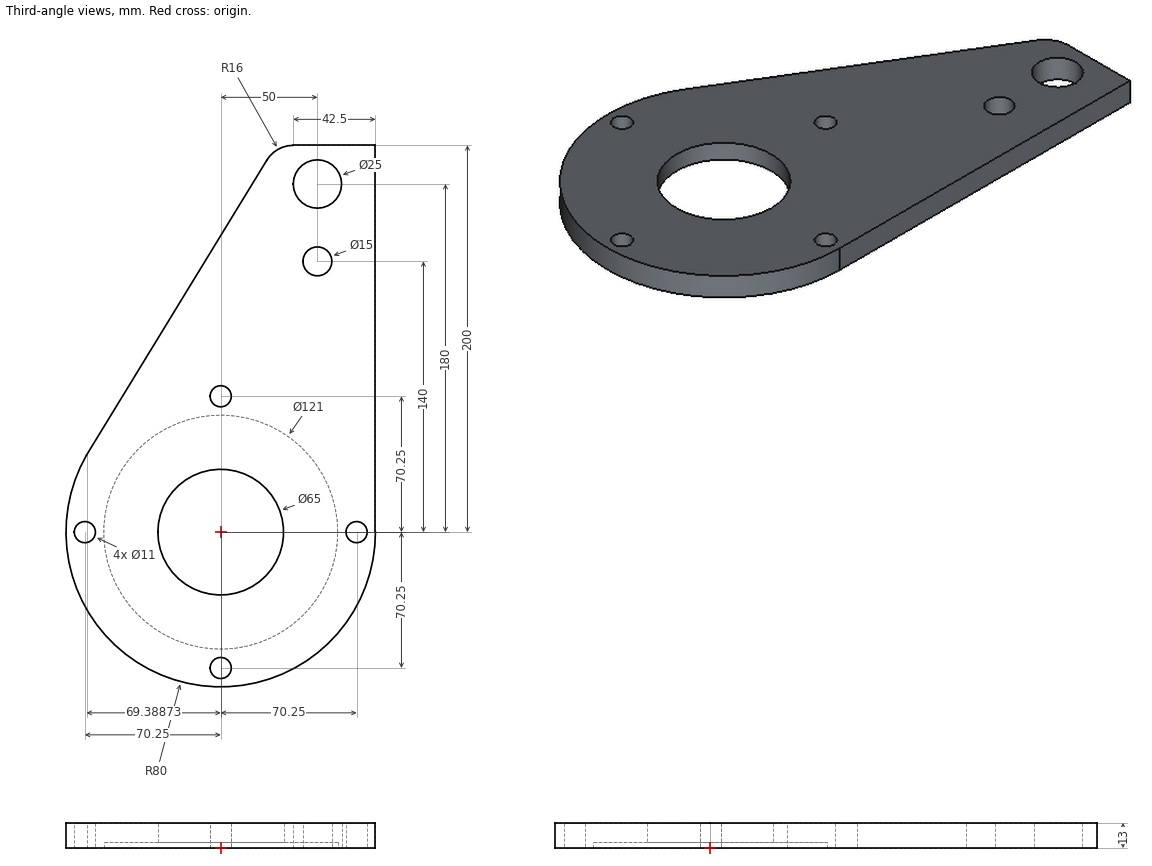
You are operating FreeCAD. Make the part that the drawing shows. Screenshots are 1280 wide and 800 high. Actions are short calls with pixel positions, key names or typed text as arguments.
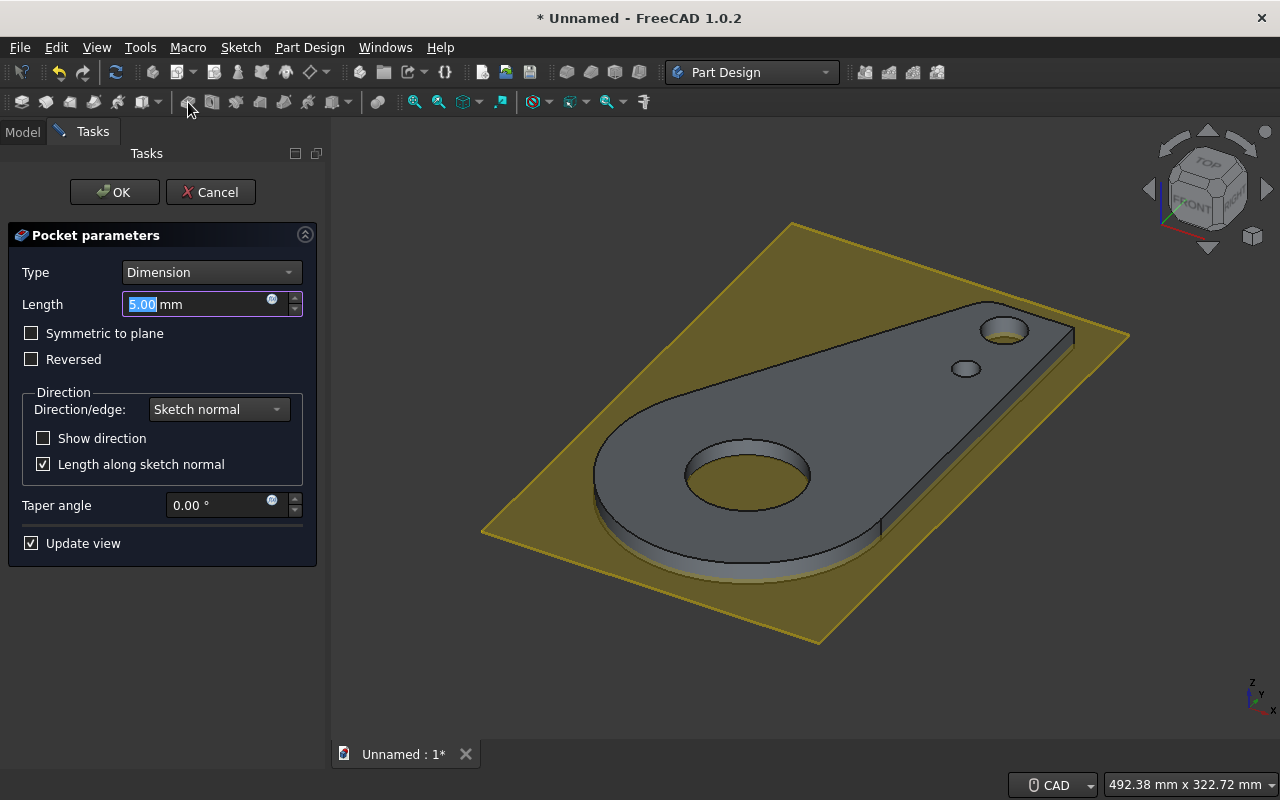
click(212, 272)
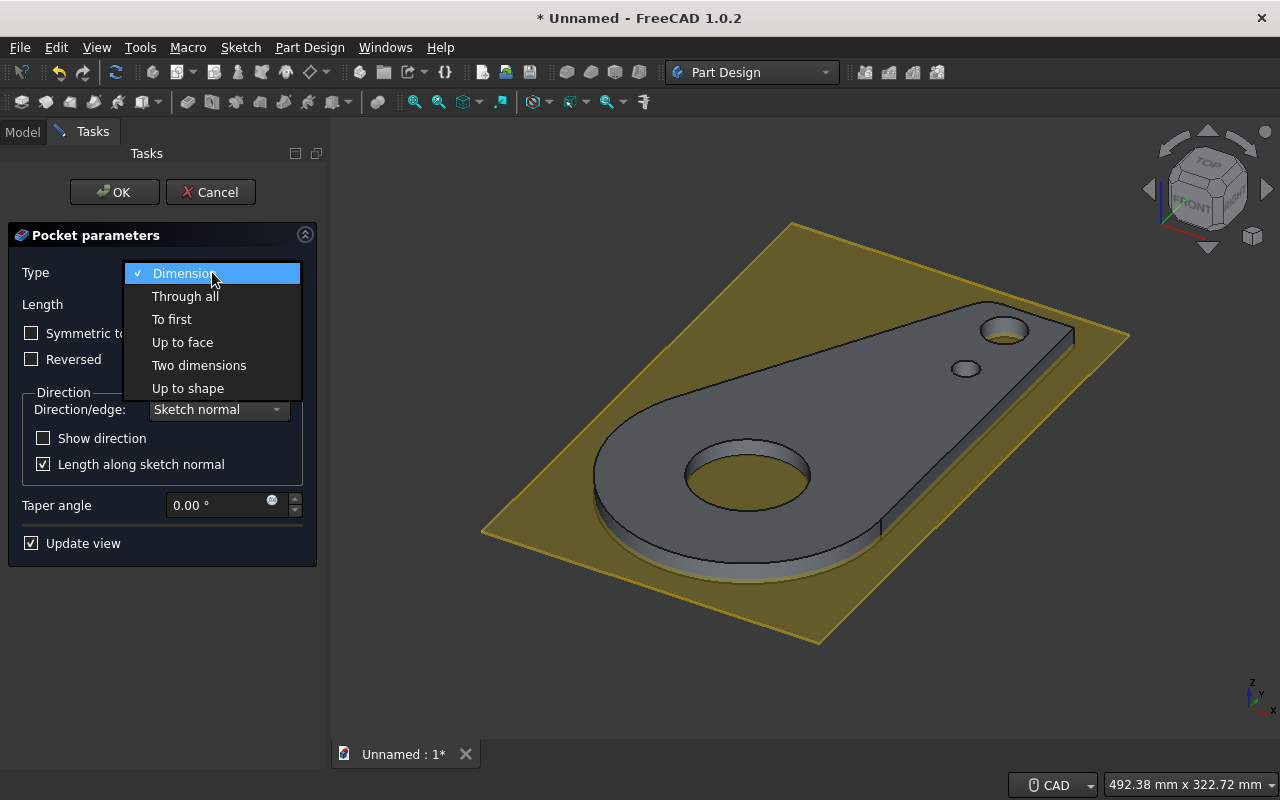
click(212, 296)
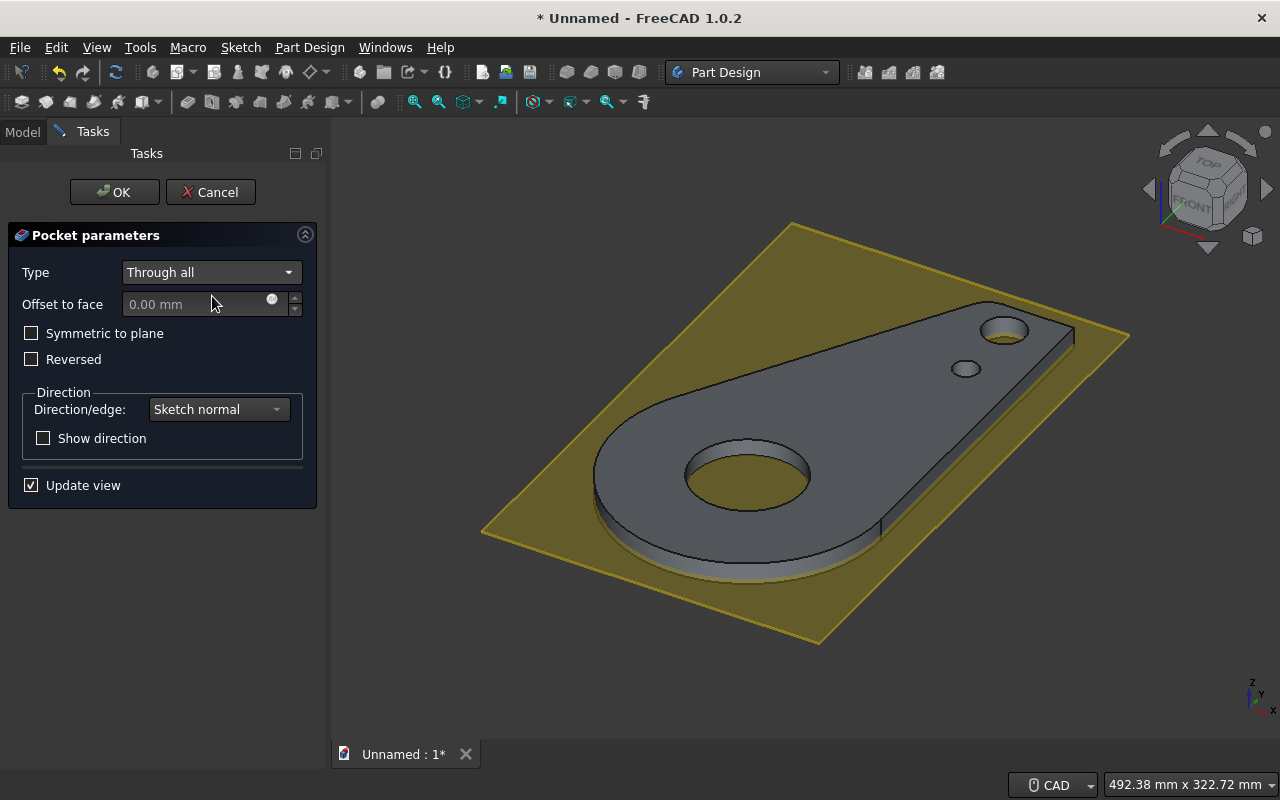
click(115, 192)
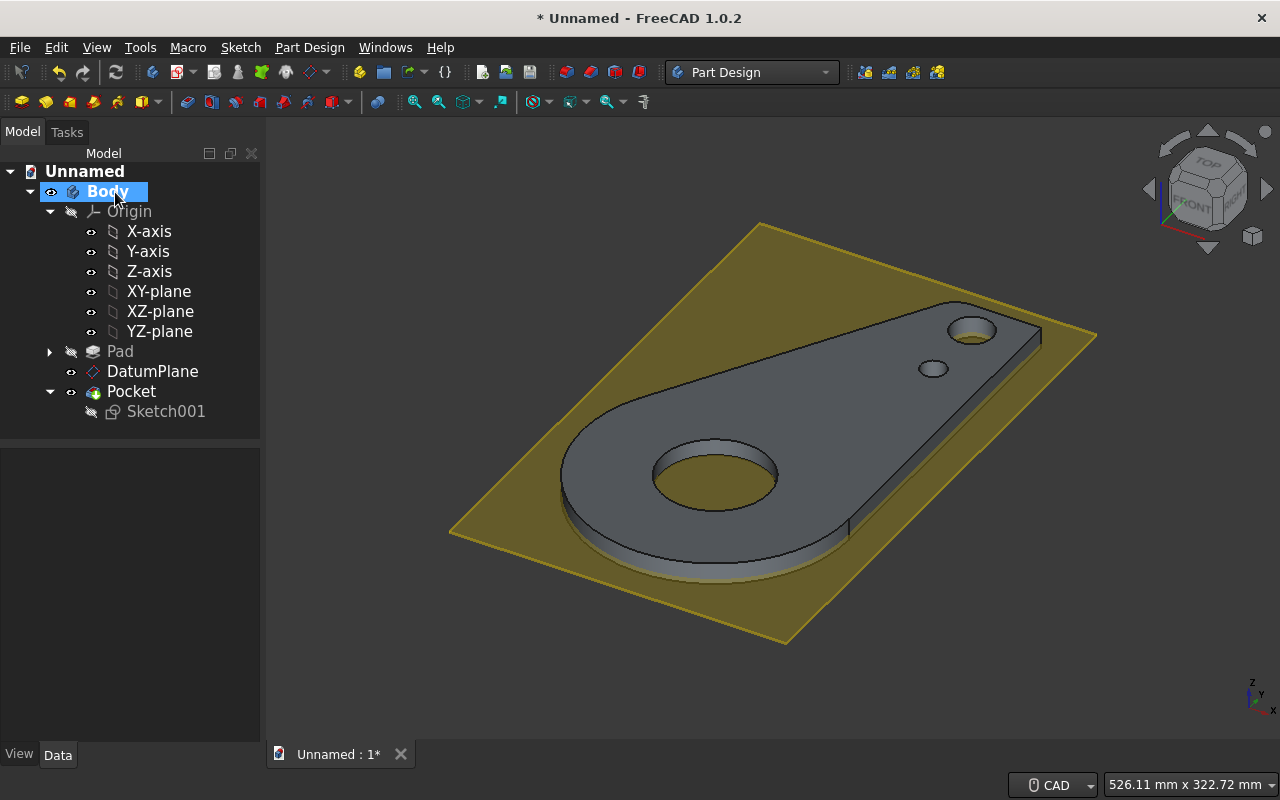
click(116, 372)
key(space)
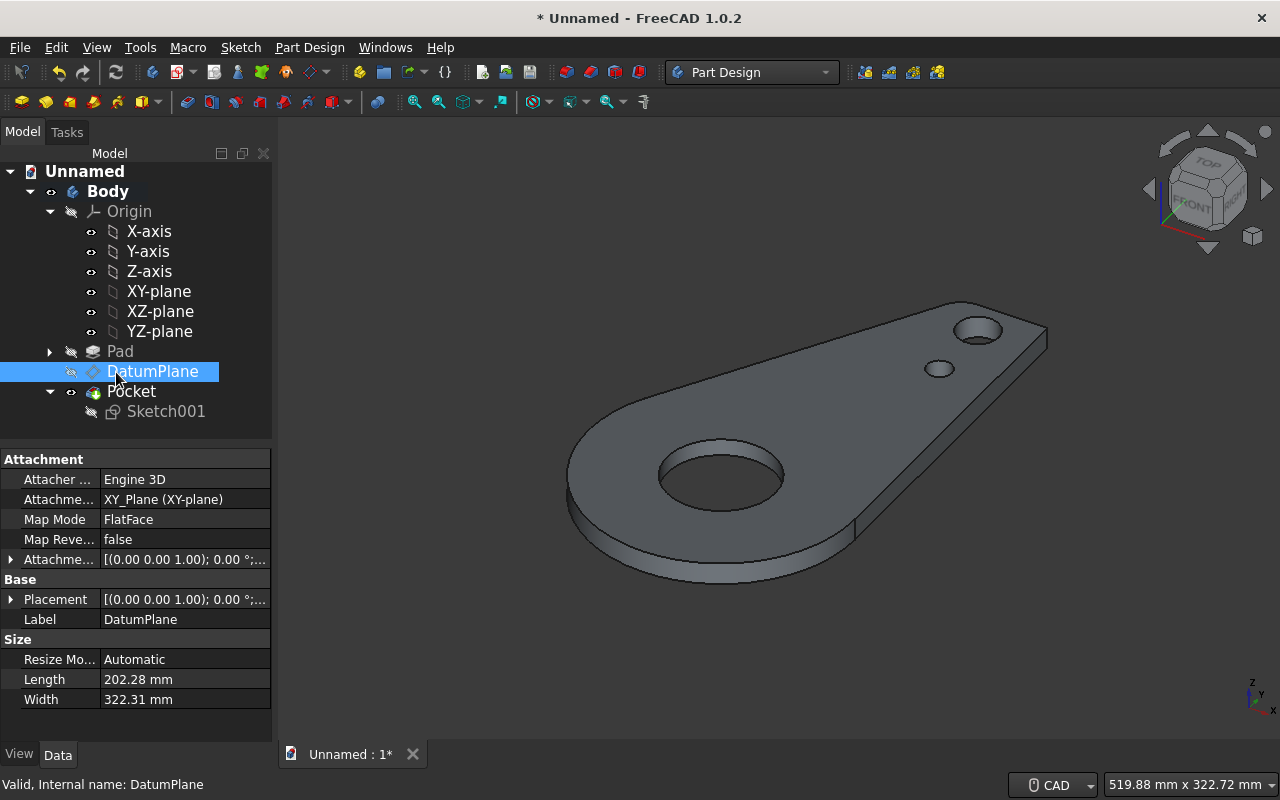
key(5)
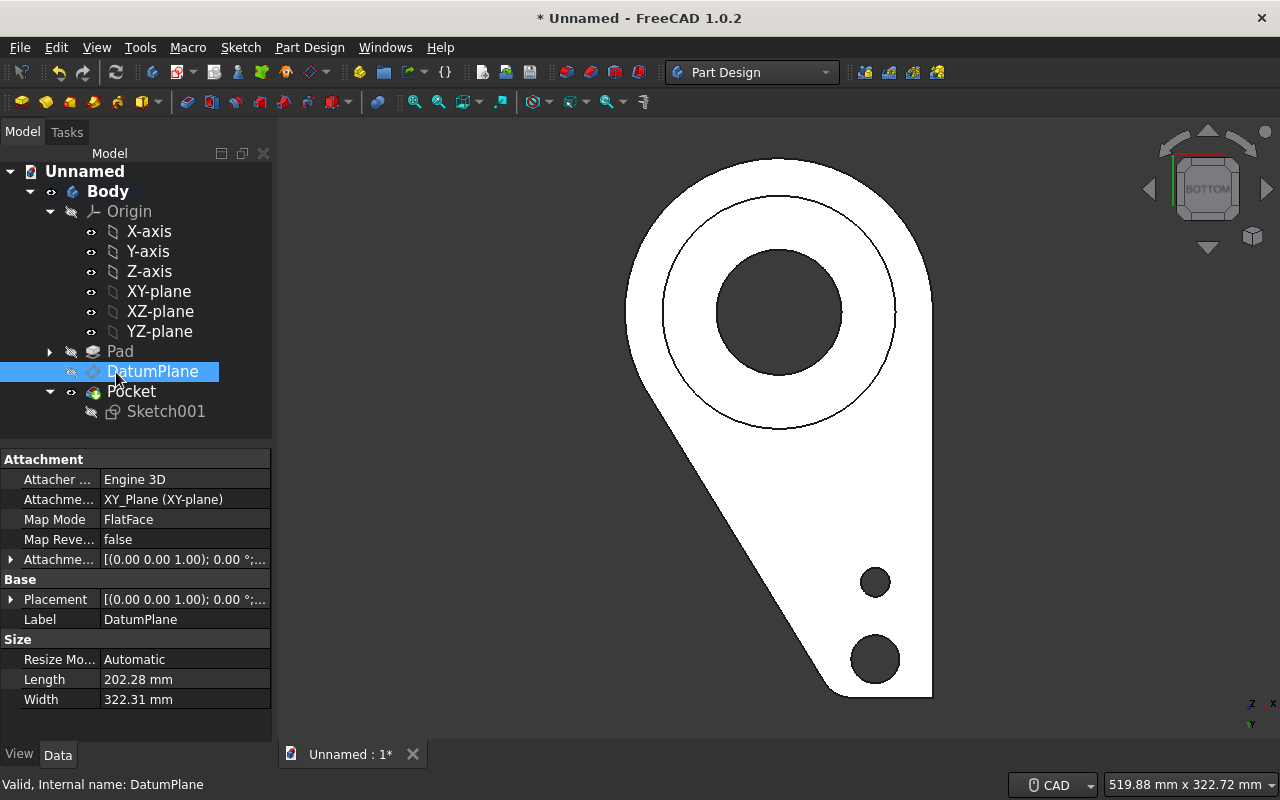
click(823, 504)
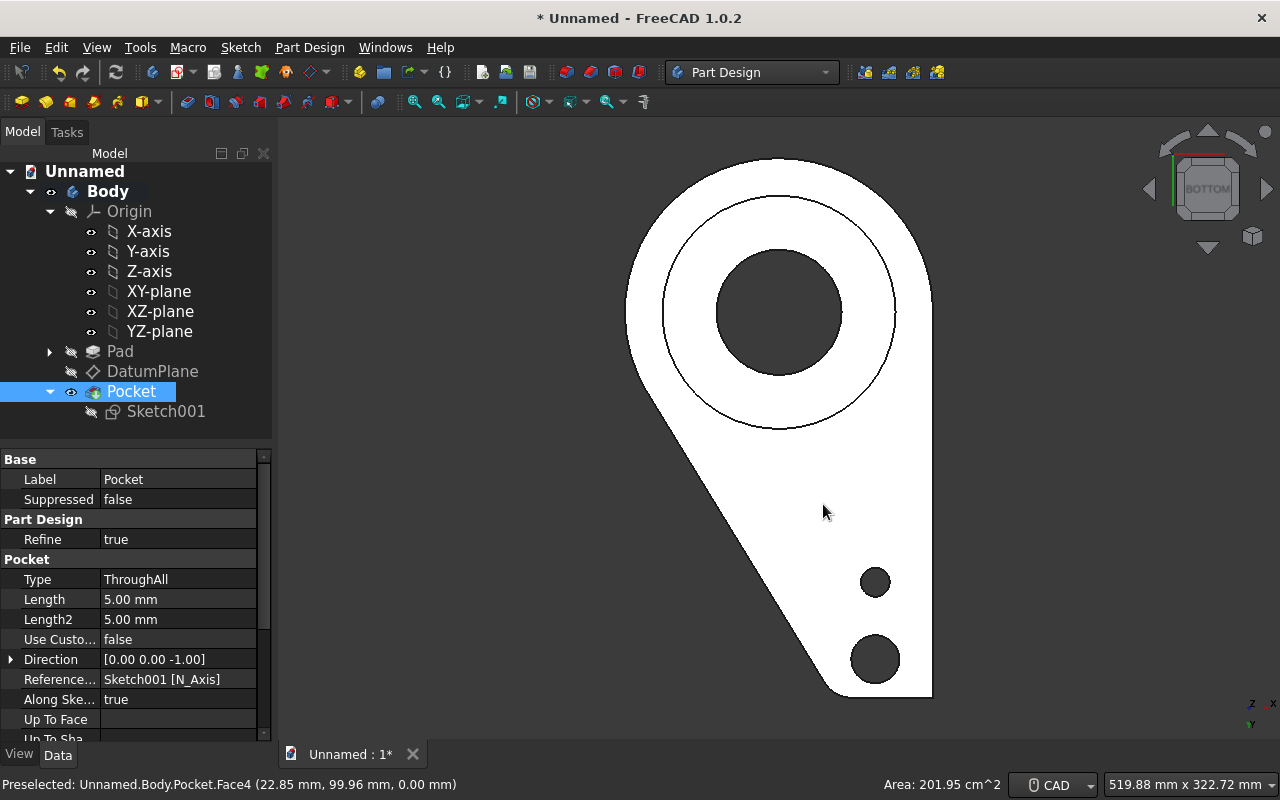
click(178, 72)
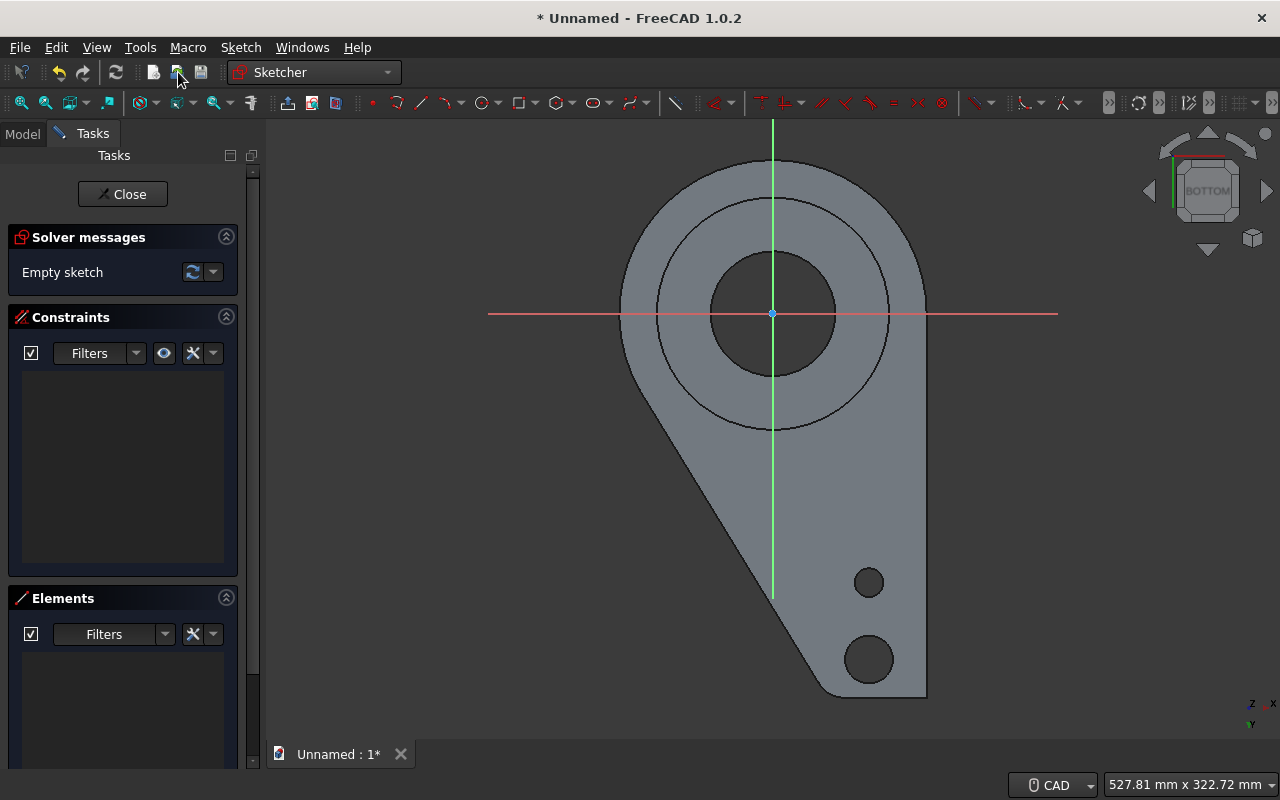
scroll(912, 147, up, 2)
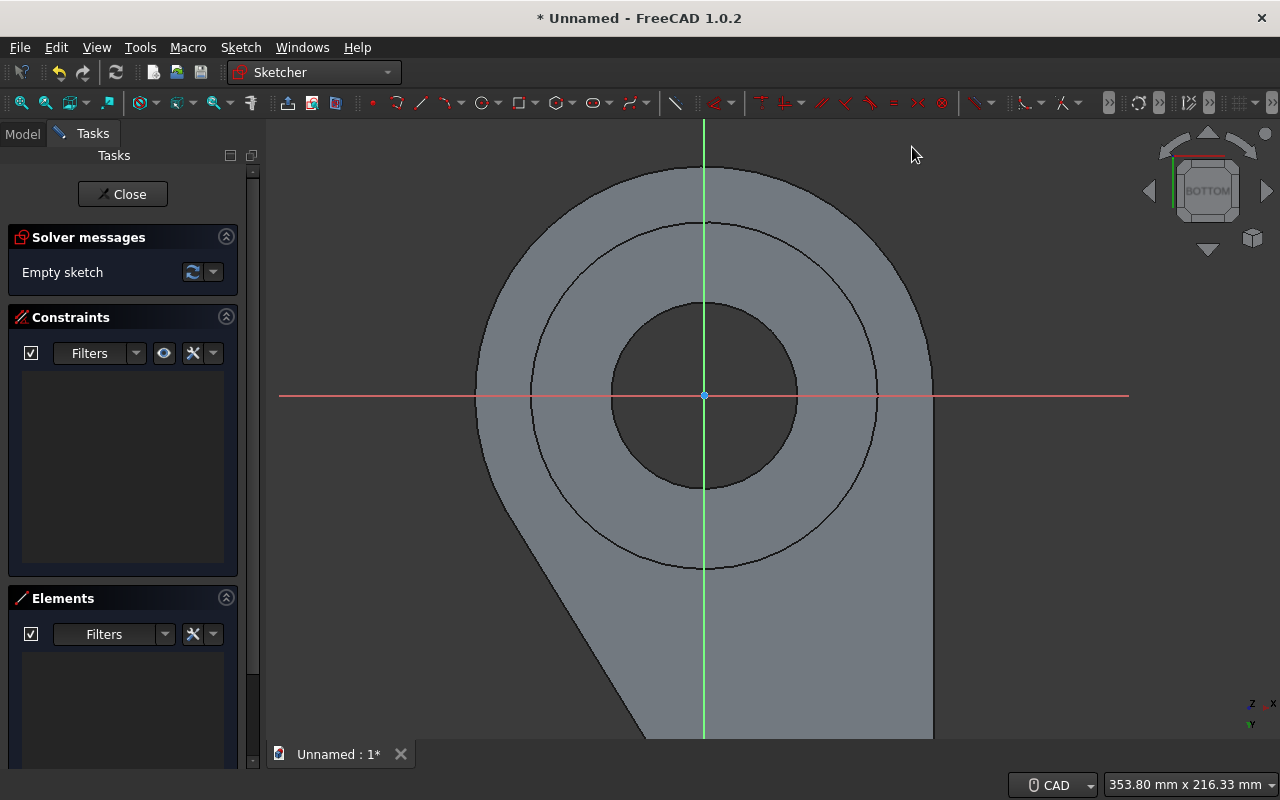
click(482, 104)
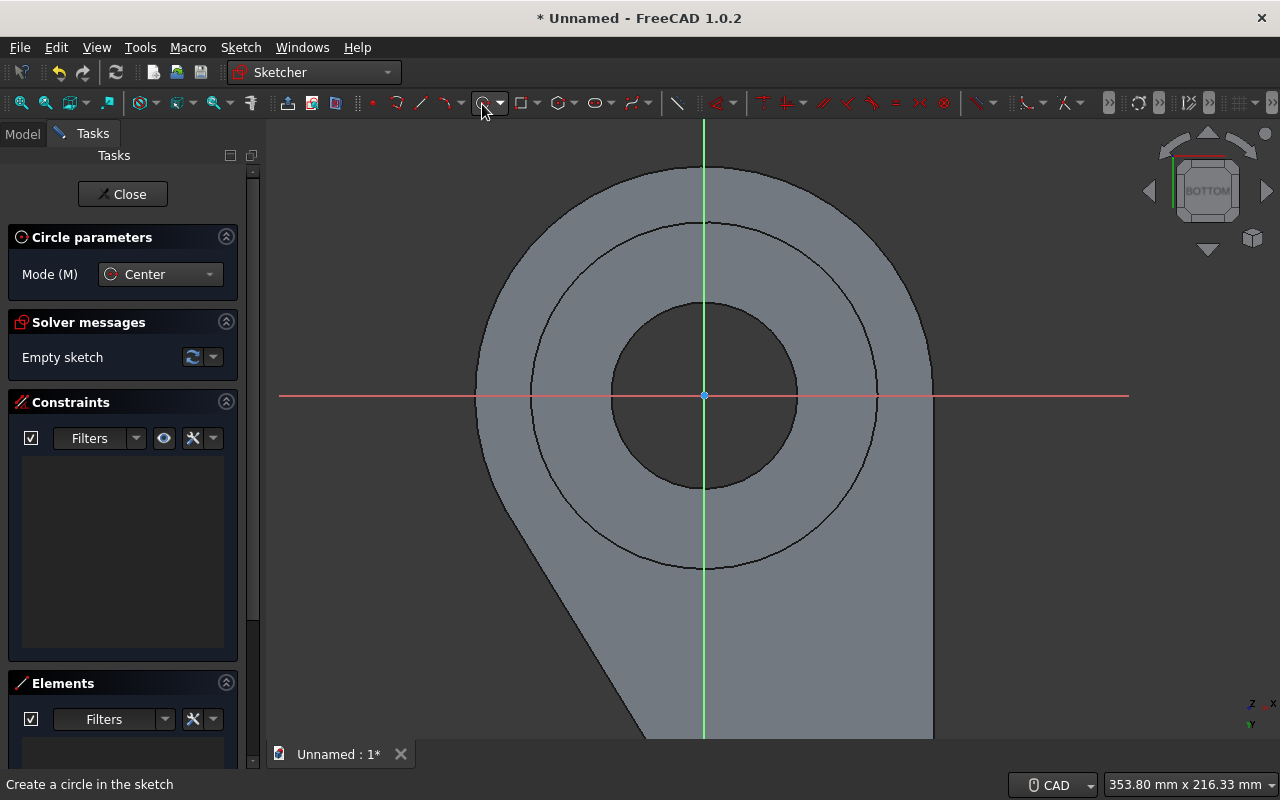
scroll(503, 396, up, 2)